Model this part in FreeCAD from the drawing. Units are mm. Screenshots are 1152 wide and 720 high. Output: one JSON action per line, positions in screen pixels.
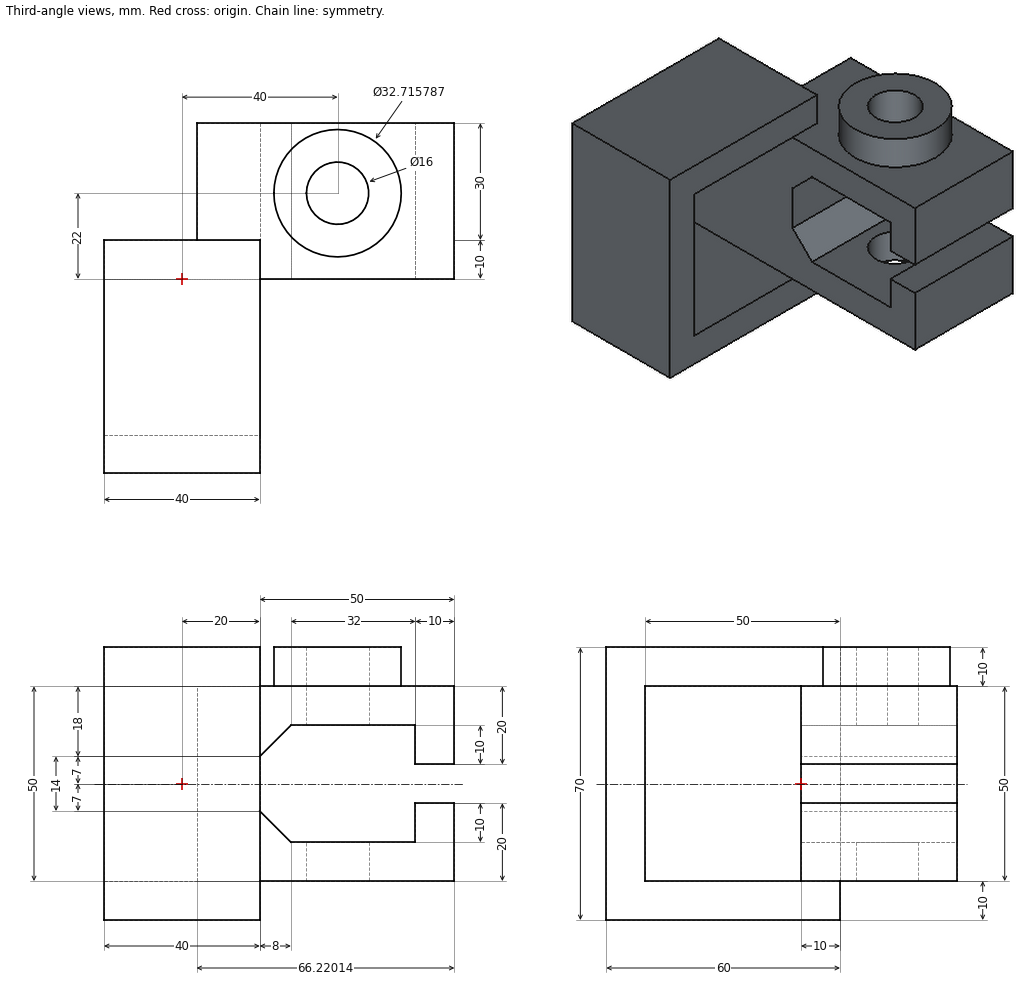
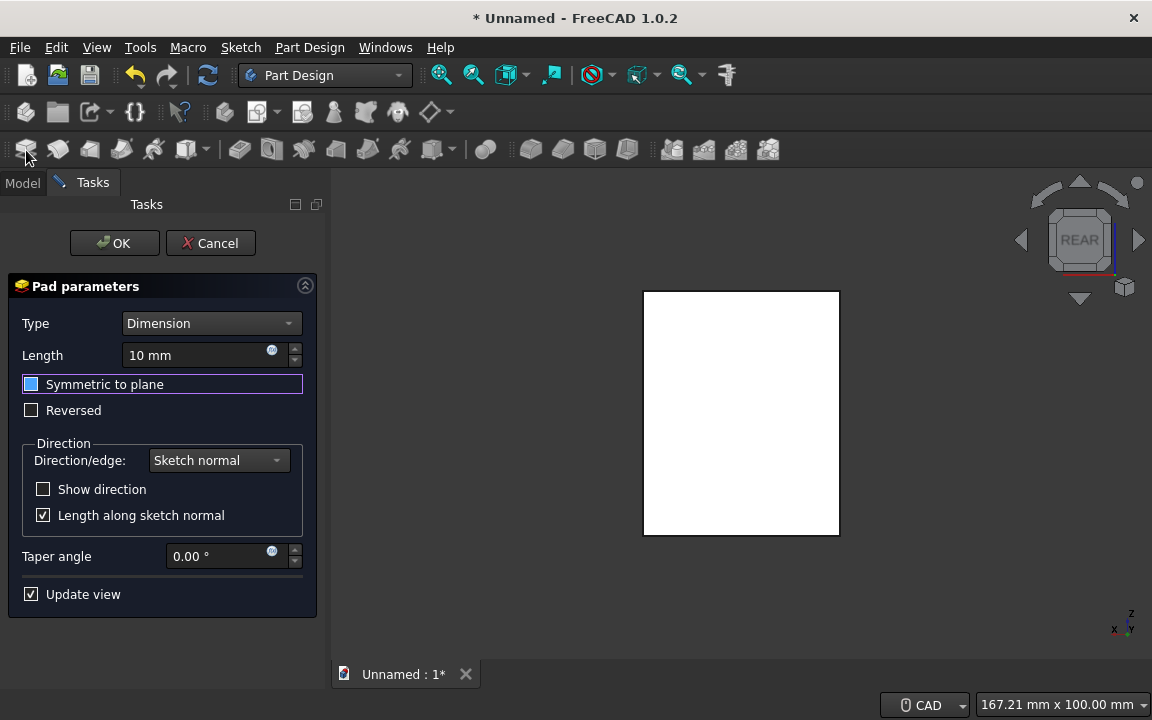
{"action": "left_click", "coordinate": [30, 410]}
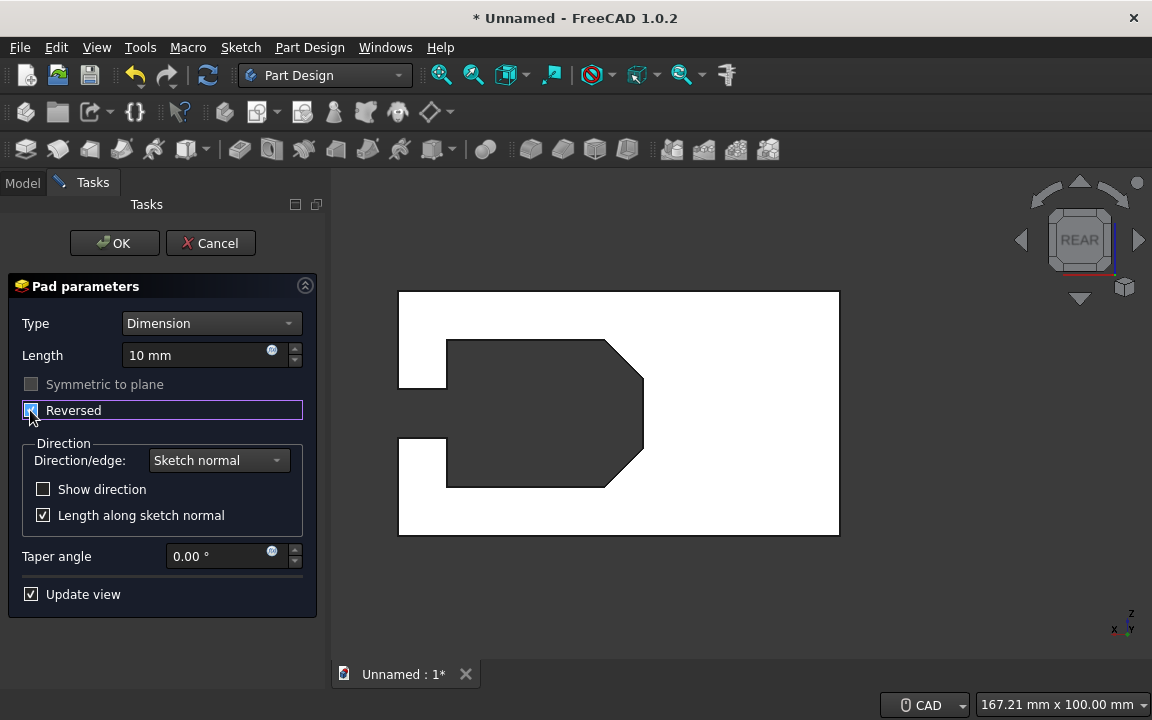
{"action": "left_click", "coordinate": [115, 243]}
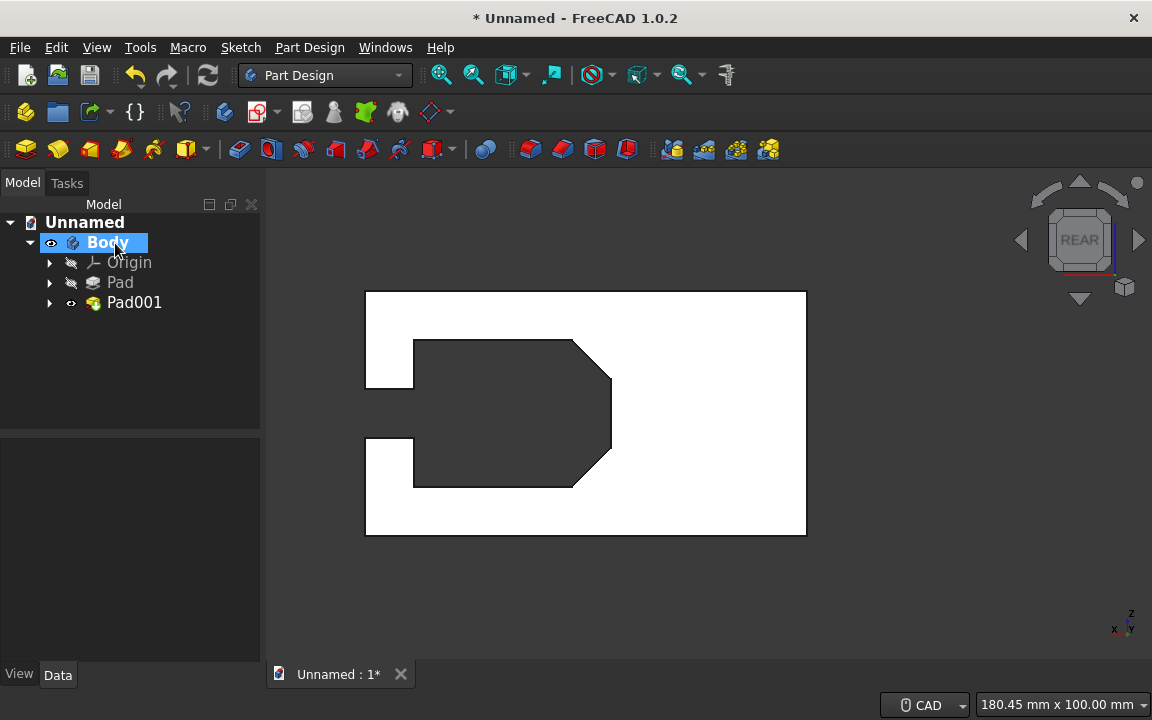
{"action": "key", "text": "6"}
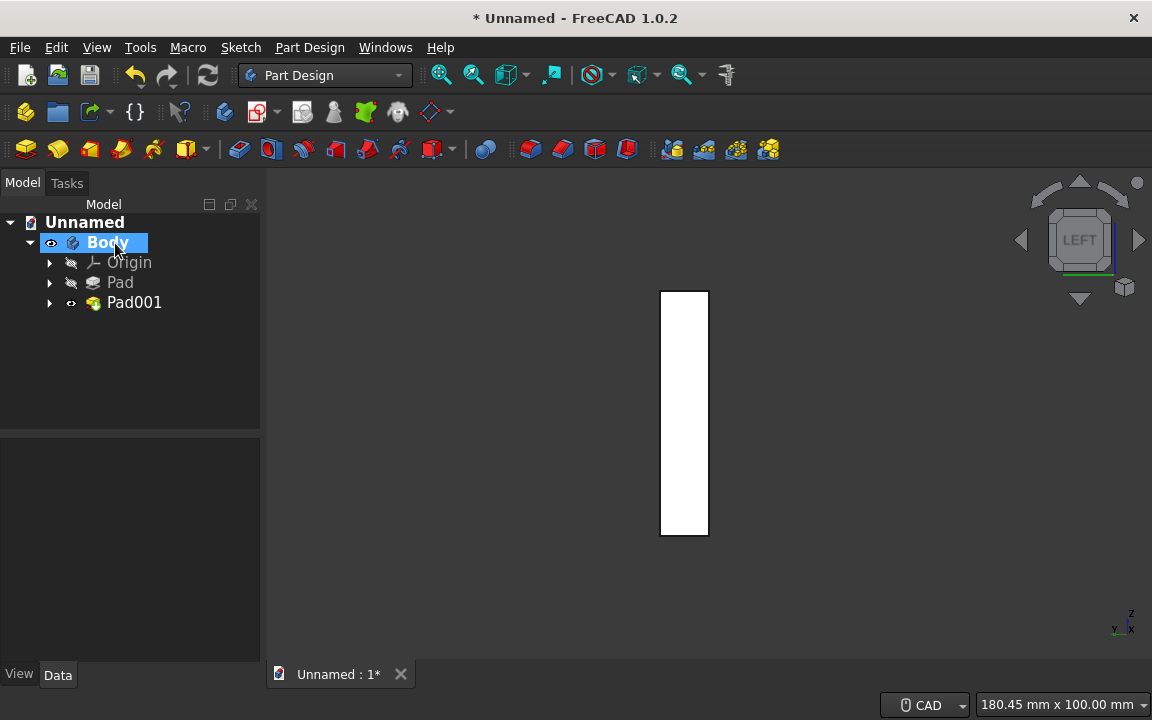
{"action": "left_click", "coordinate": [684, 413]}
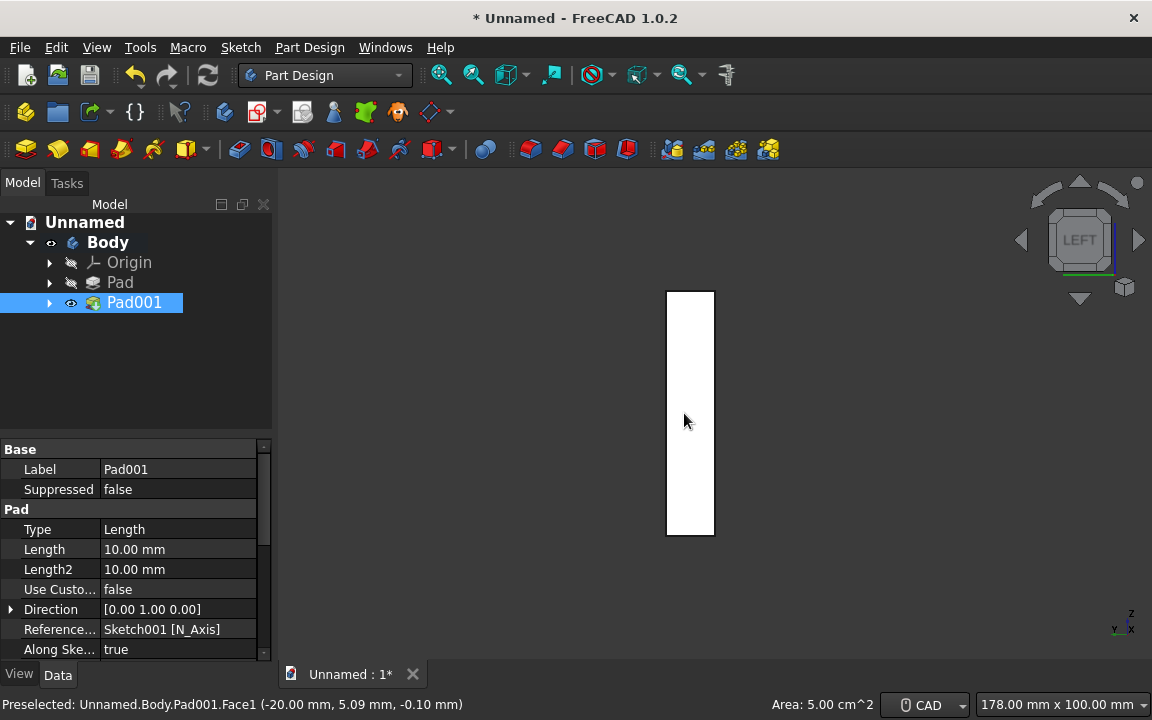
{"action": "left_click", "coordinate": [258, 112]}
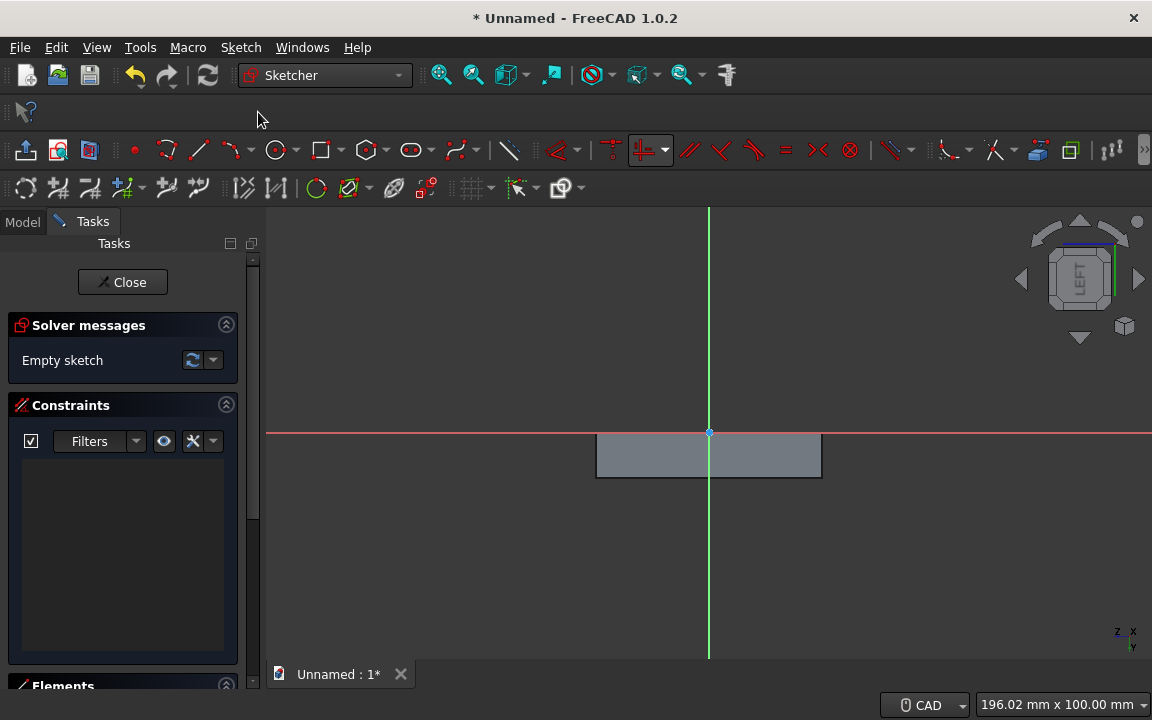
{"action": "scroll", "coordinate": [331, 631], "scroll_direction": "down", "scroll_amount": 1}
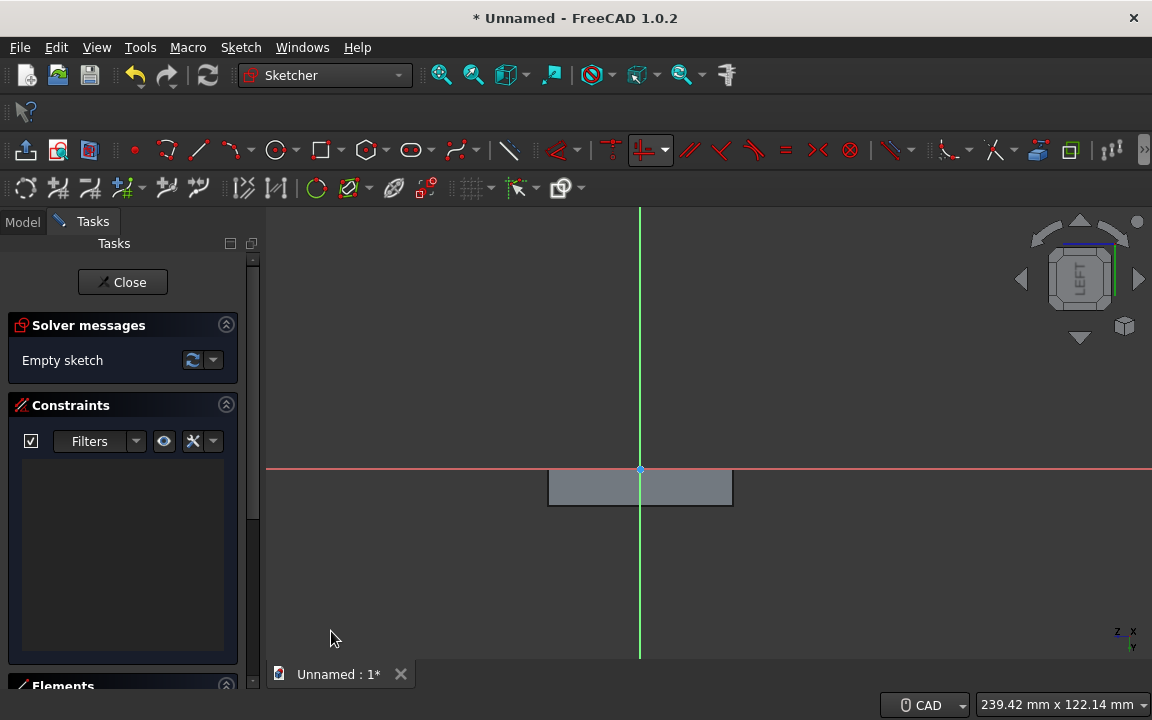
{"action": "key", "text": "g m"}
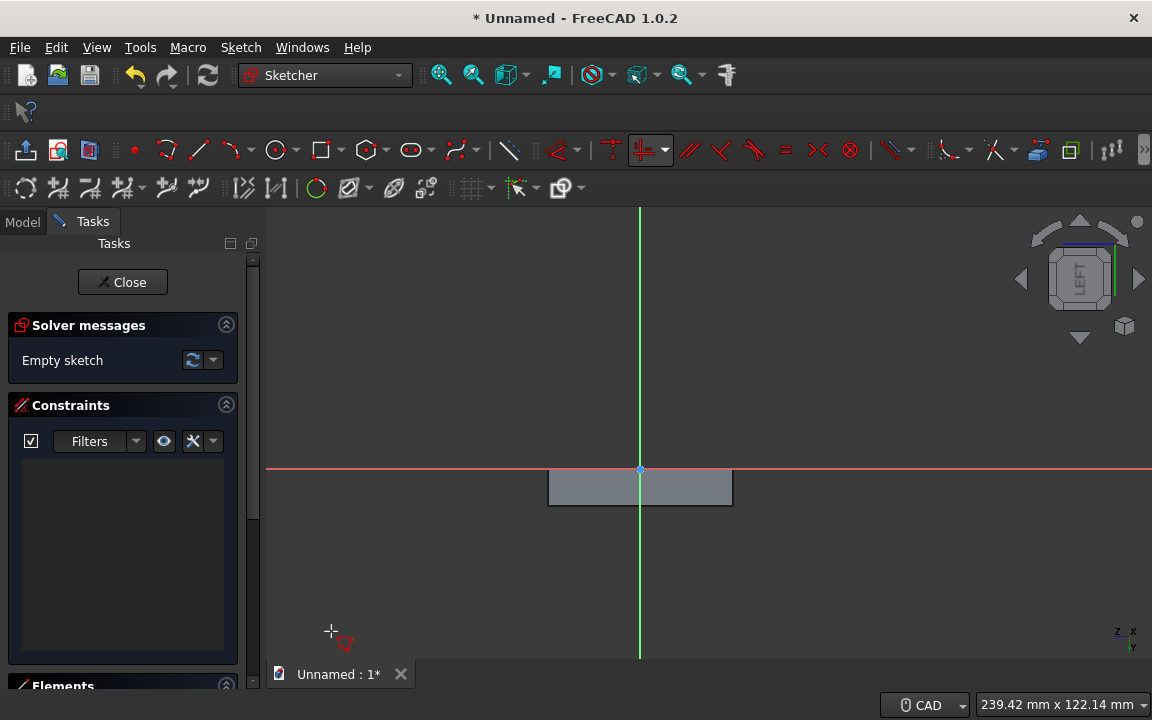
{"action": "left_click", "coordinate": [733, 506]}
{"action": "left_click", "coordinate": [770, 506]}
{"action": "left_click", "coordinate": [770, 284]}
{"action": "left_click", "coordinate": [511, 284]}
{"action": "left_click", "coordinate": [511, 506]}
{"action": "left_click", "coordinate": [548, 506]}
{"action": "left_click", "coordinate": [548, 321]}
{"action": "left_click", "coordinate": [733, 321]}
{"action": "left_click", "coordinate": [733, 507]}
{"action": "key", "text": "Escape"}
{"action": "key", "text": "Escape"}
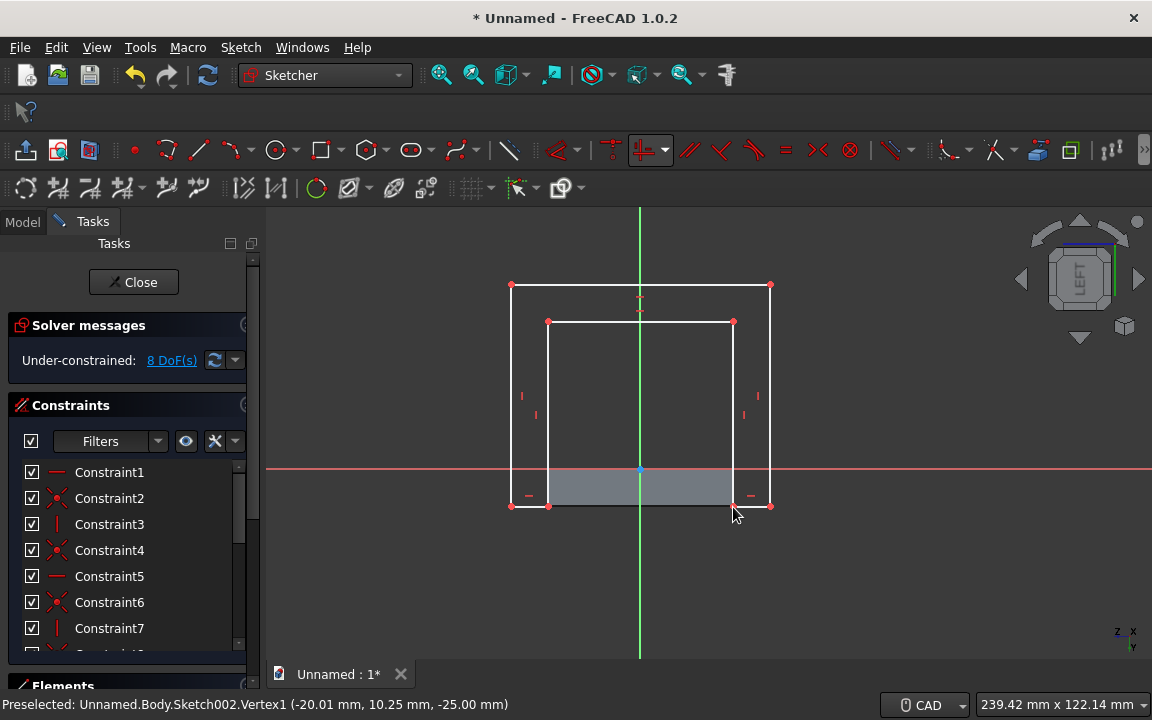
{"action": "left_click", "coordinate": [770, 507]}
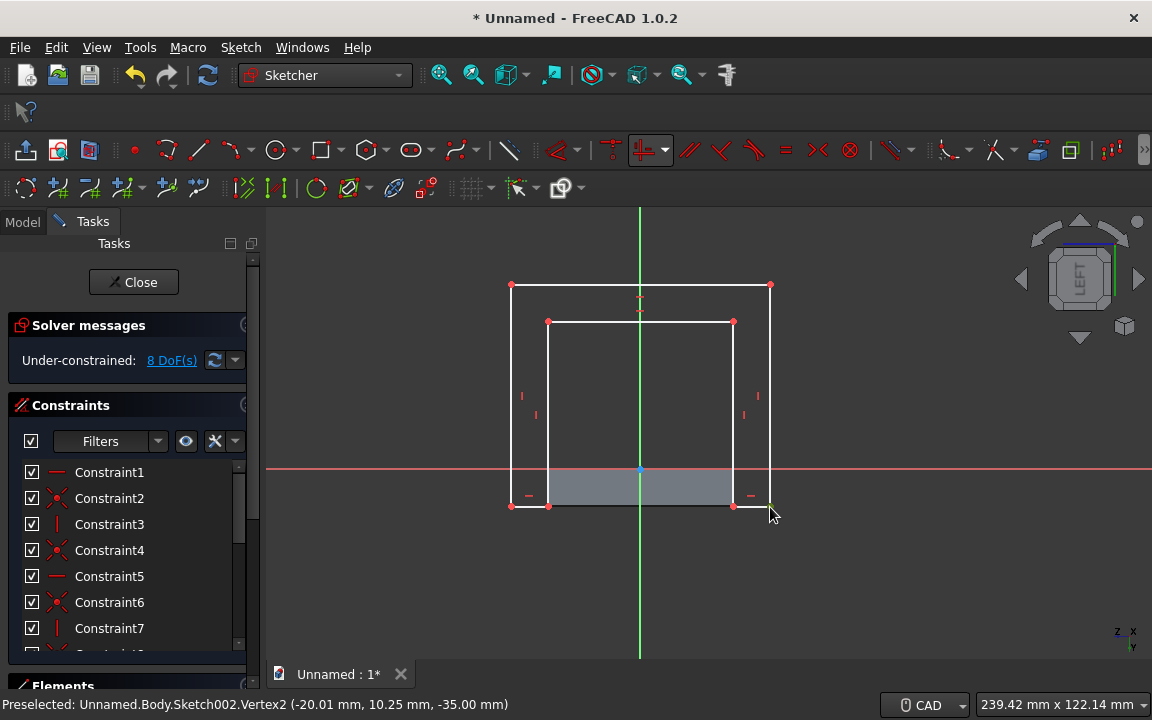
{"action": "left_click", "coordinate": [511, 507]}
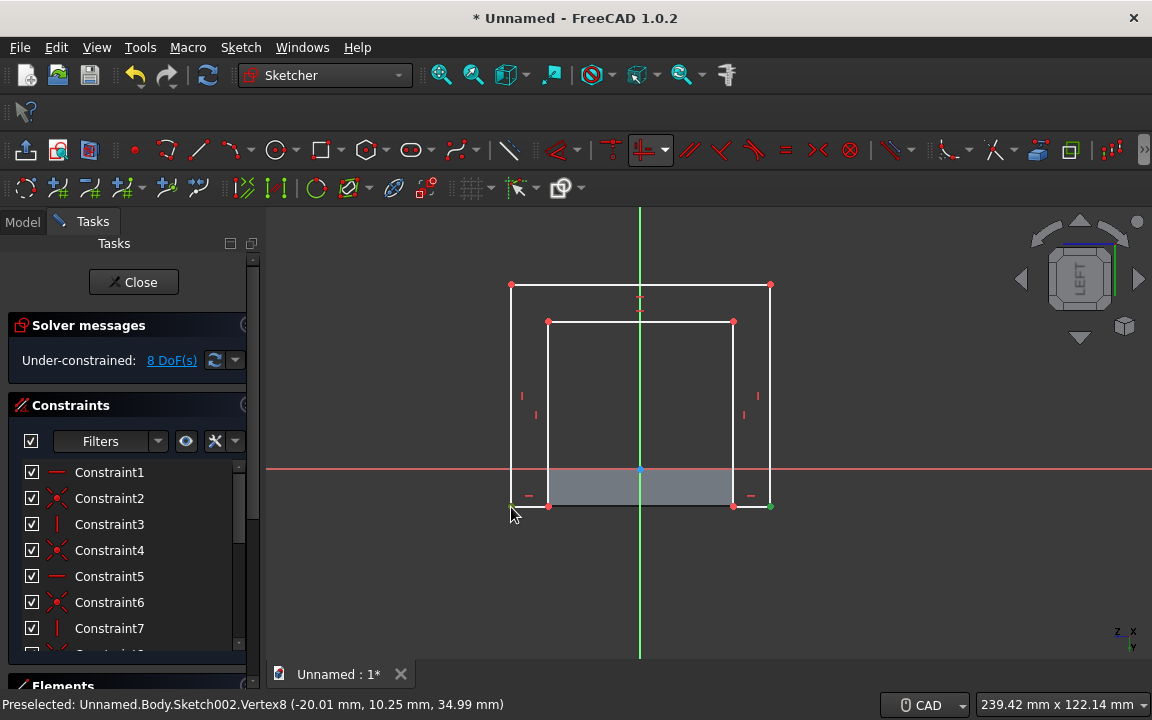
{"action": "left_click", "coordinate": [640, 603]}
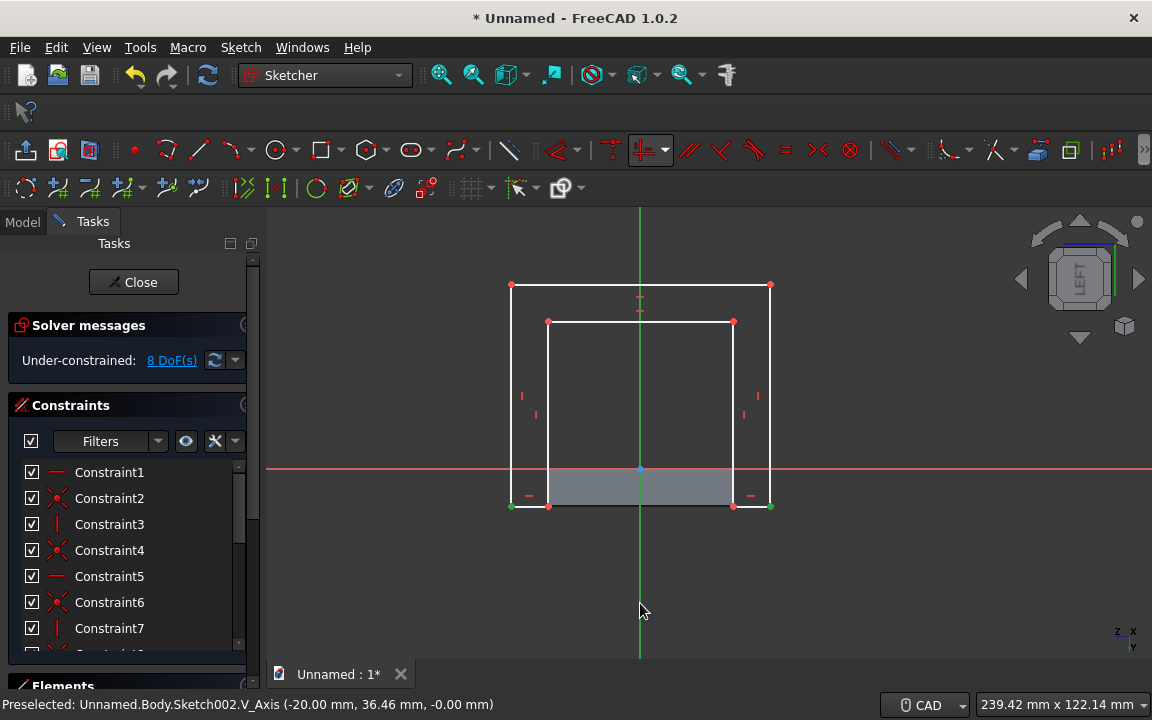
{"action": "key", "text": "s"}